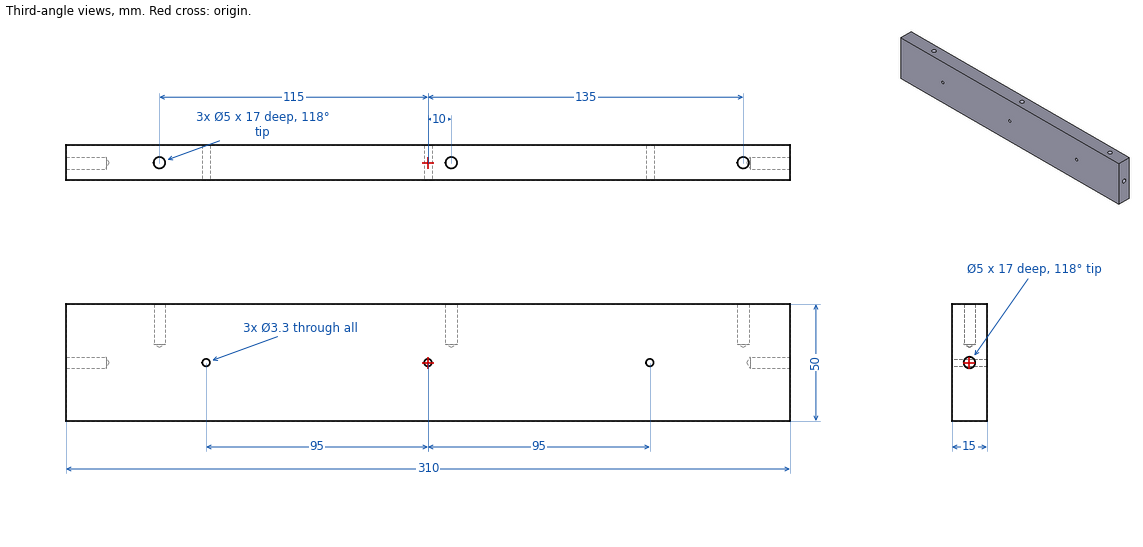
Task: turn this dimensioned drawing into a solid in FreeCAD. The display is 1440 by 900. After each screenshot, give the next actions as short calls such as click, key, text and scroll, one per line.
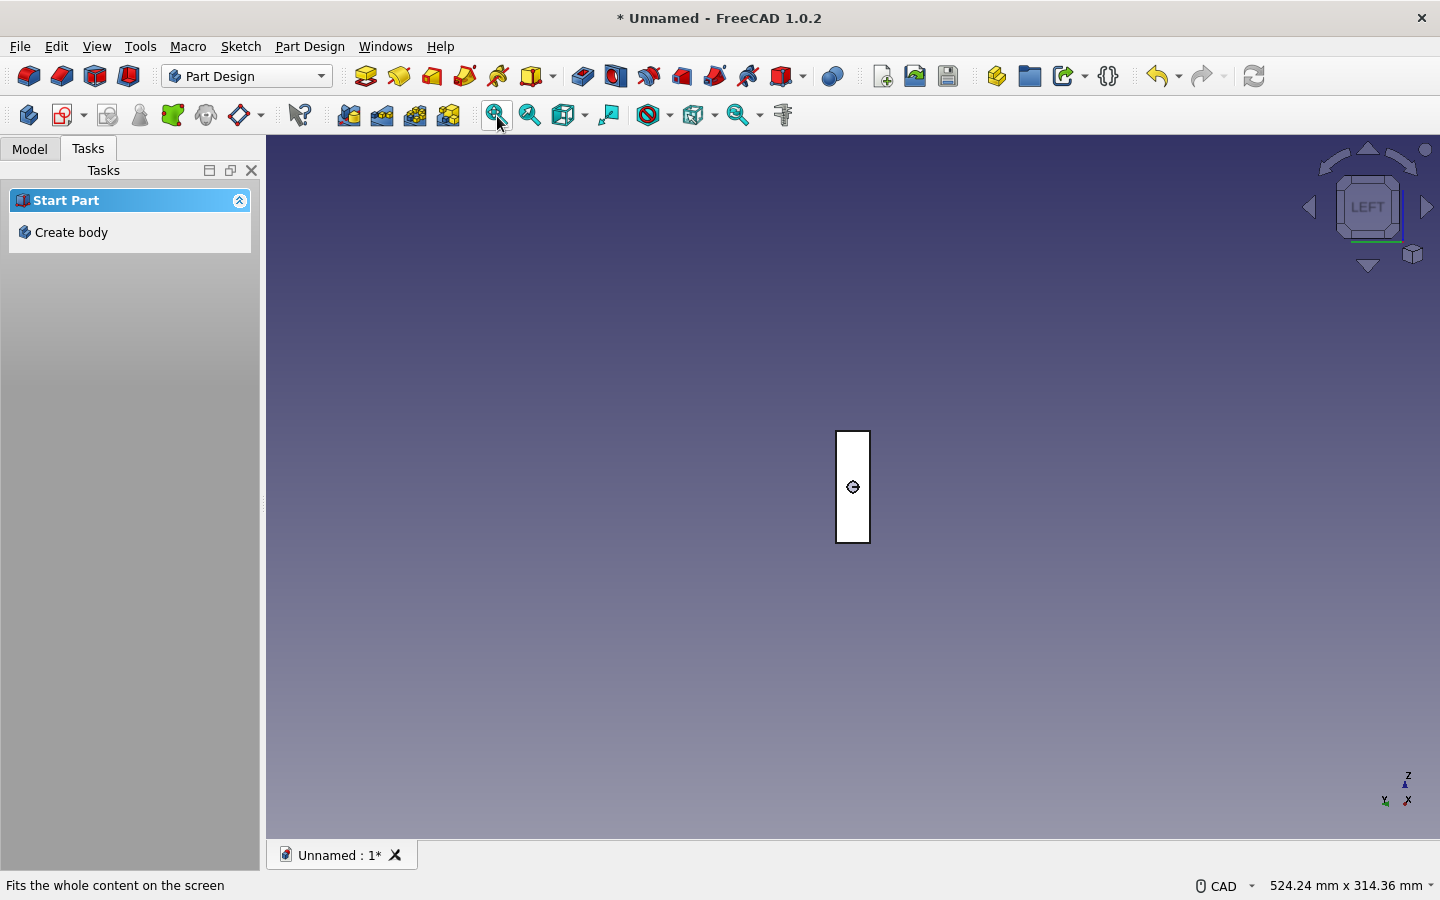
key(4)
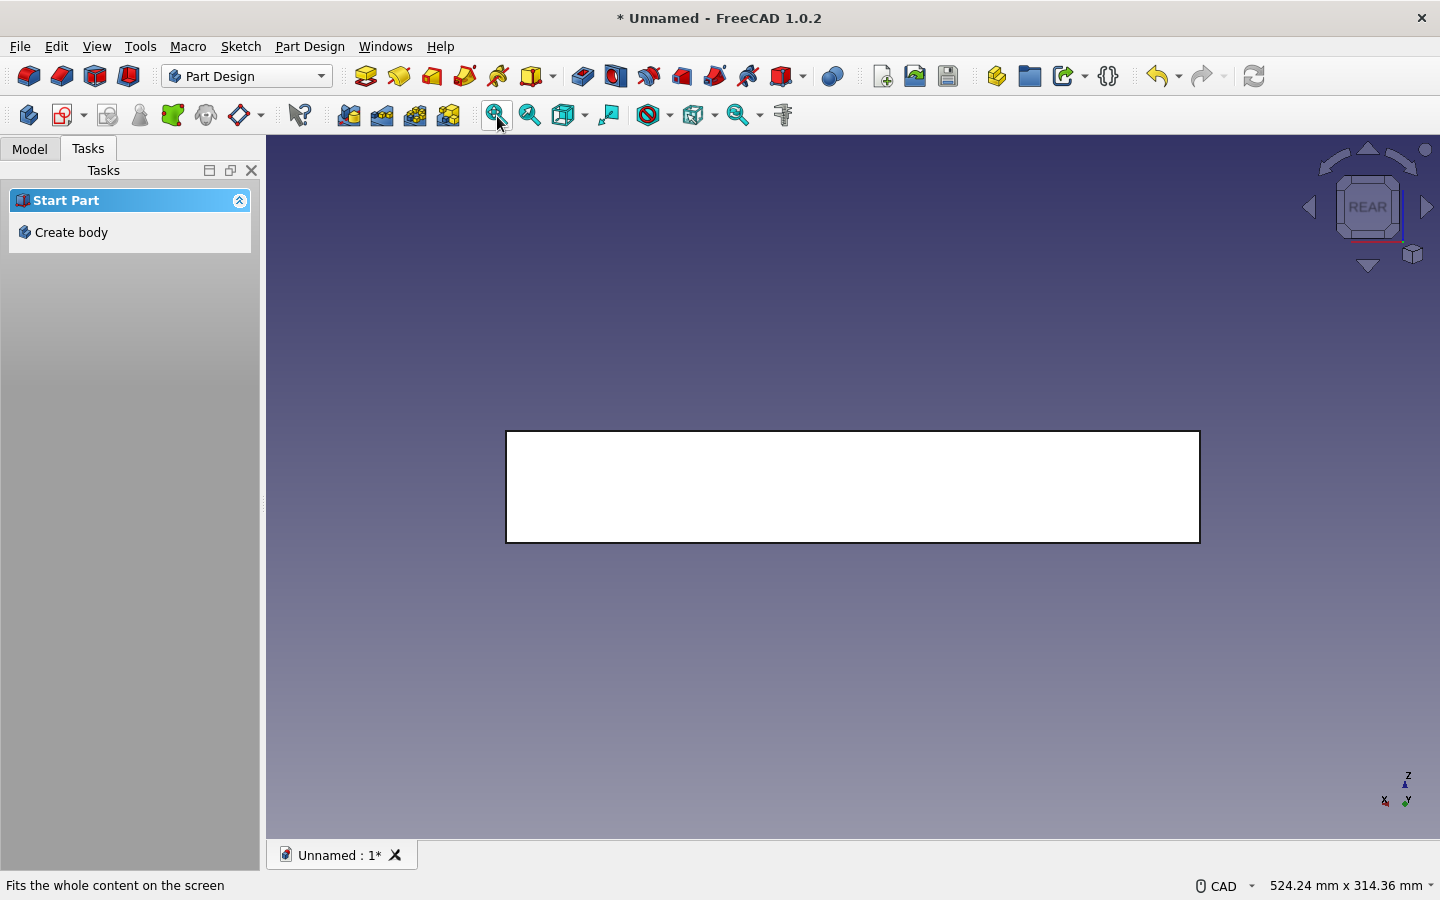
click(655, 486)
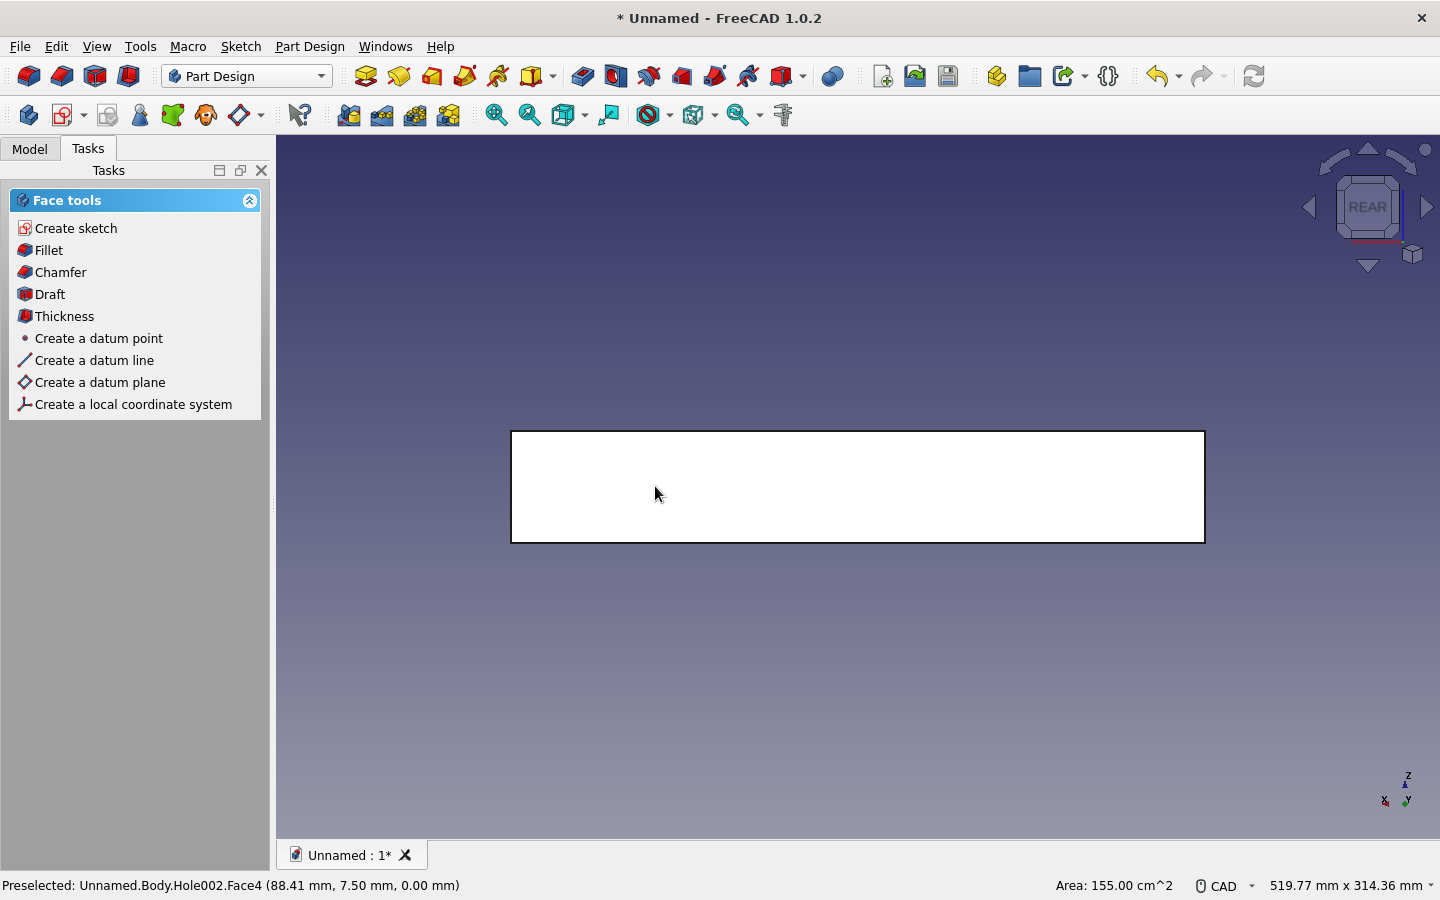
click(62, 116)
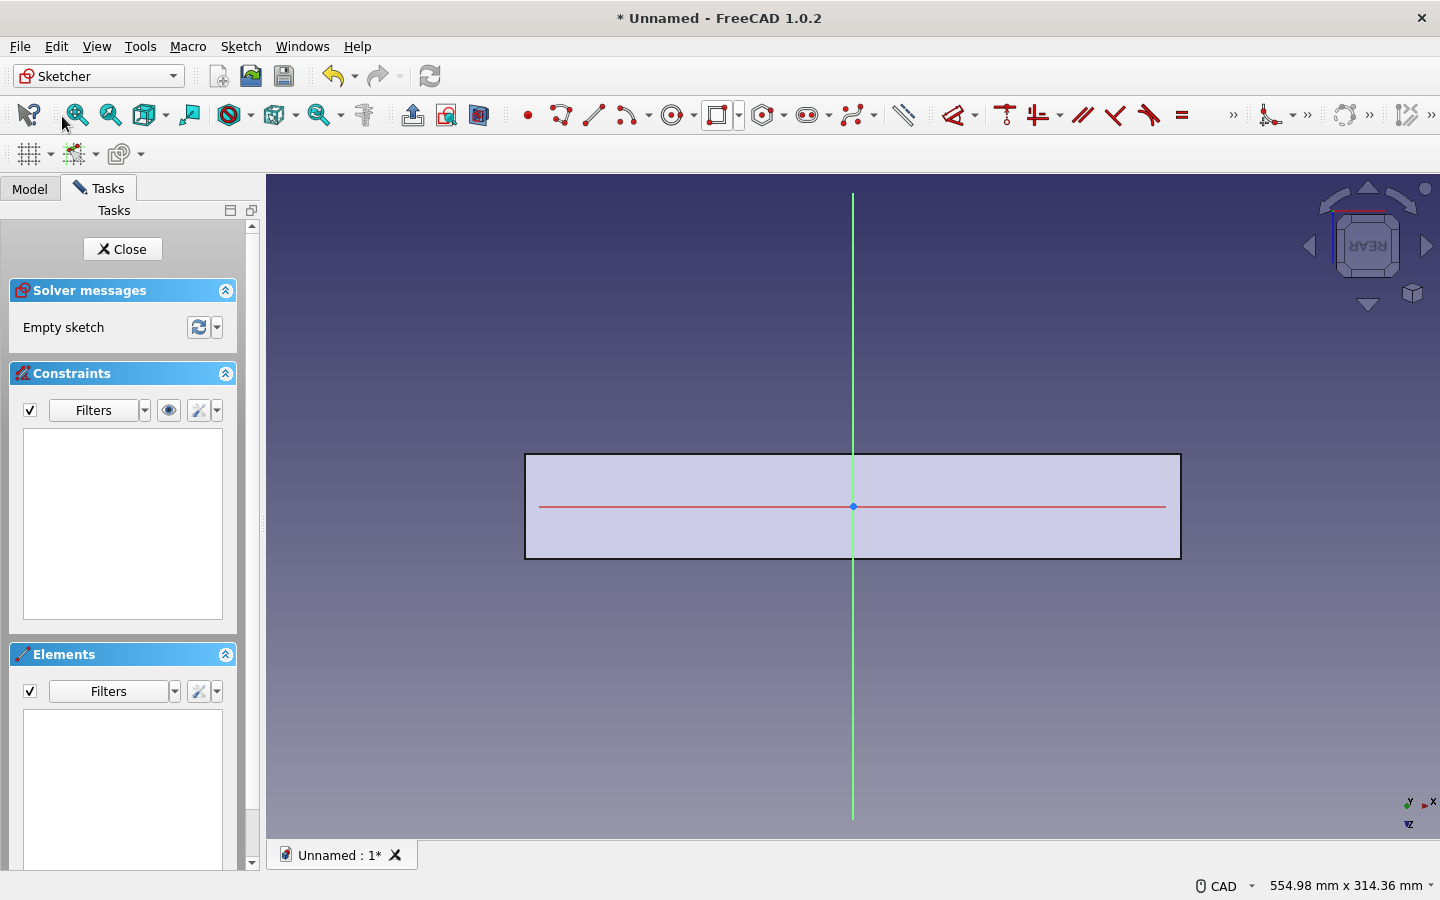
scroll(936, 507, up, 3)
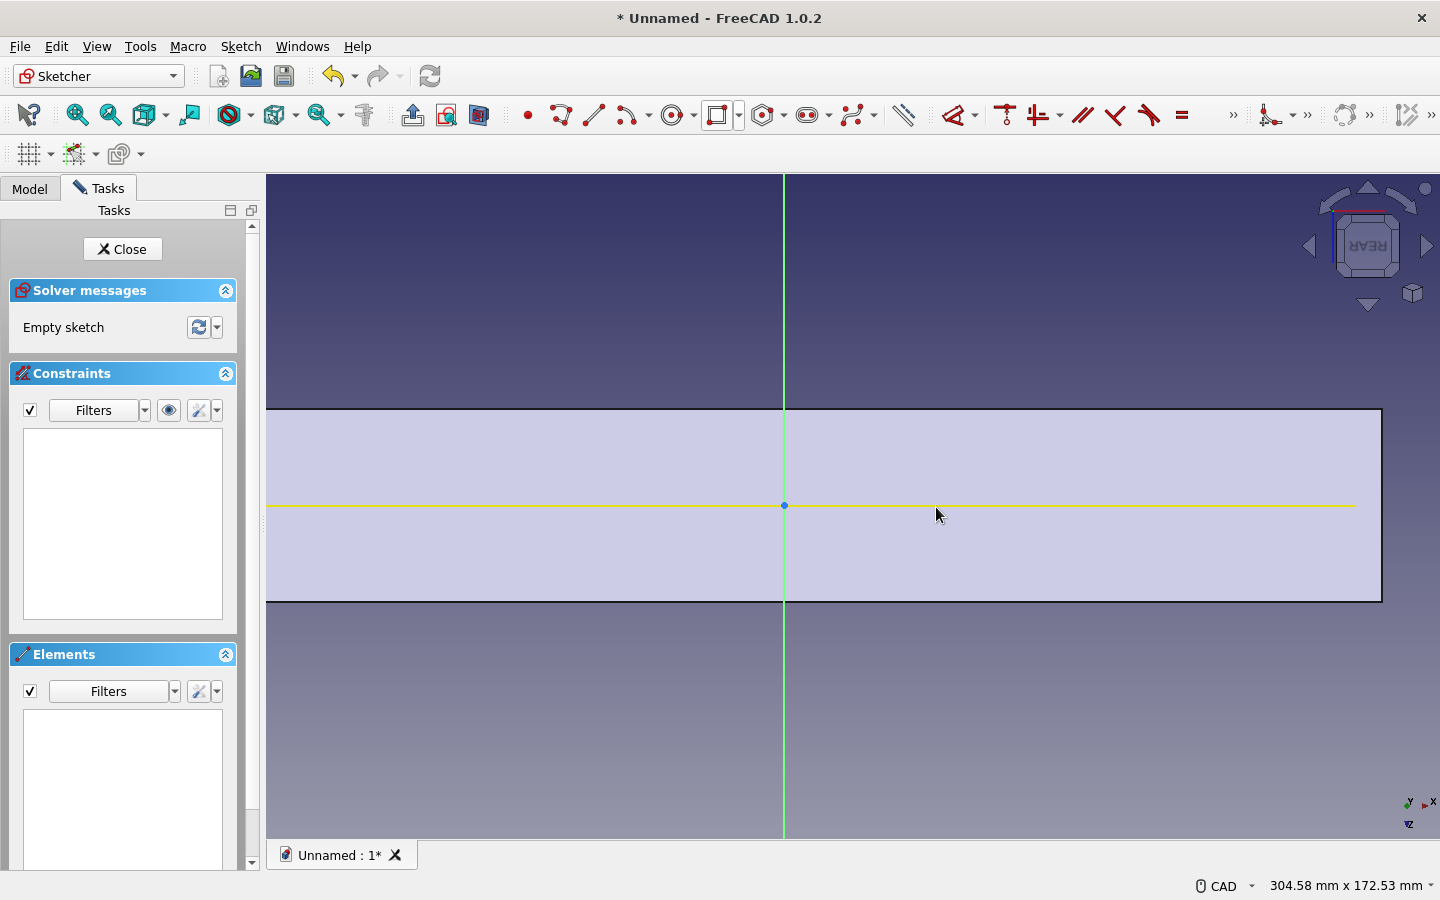
click(672, 116)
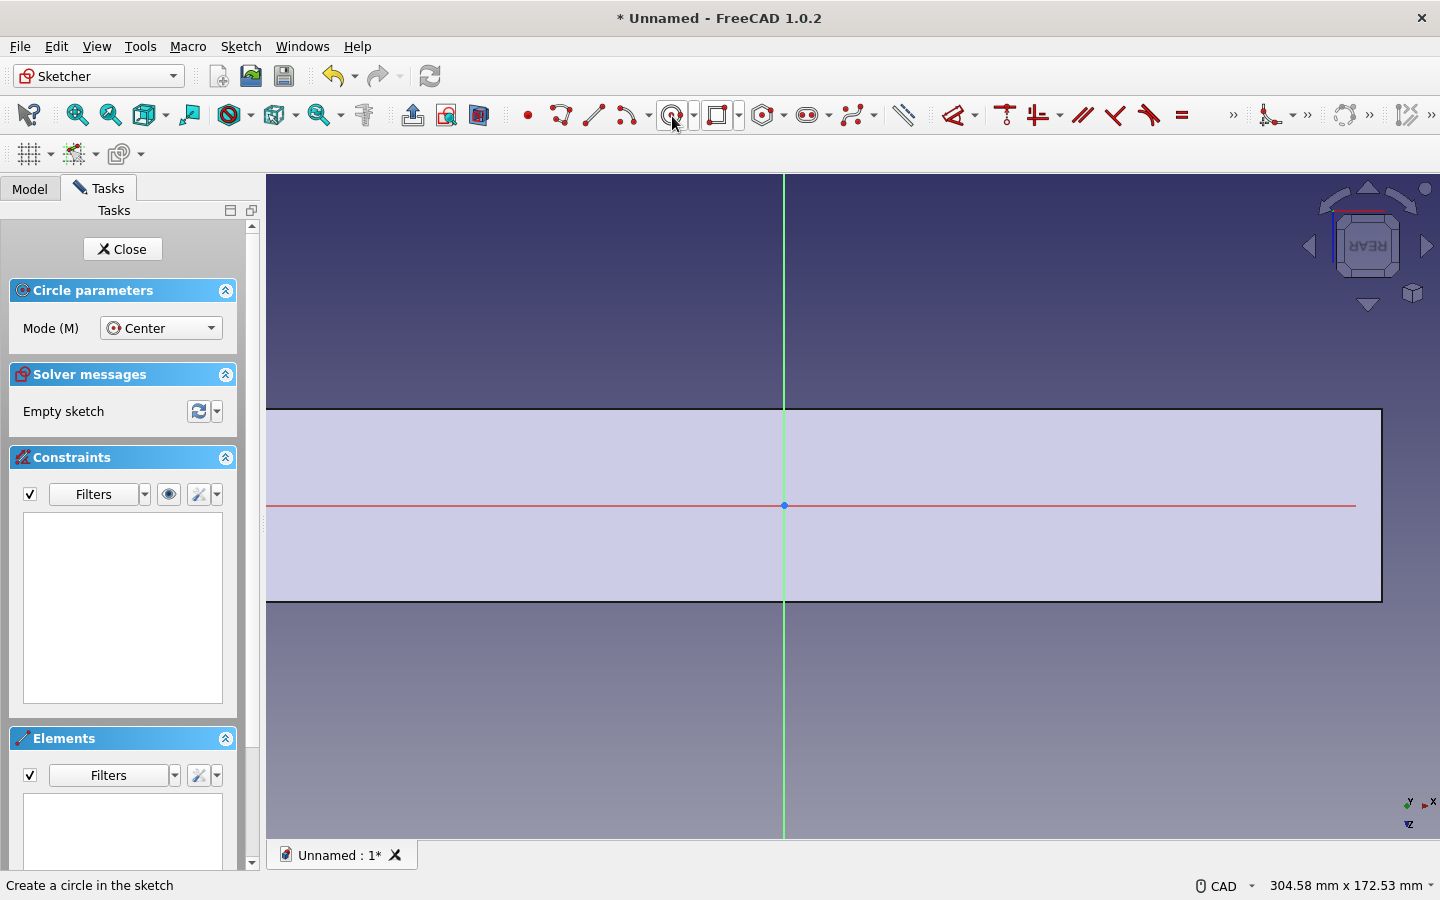
scroll(418, 506, up, 7)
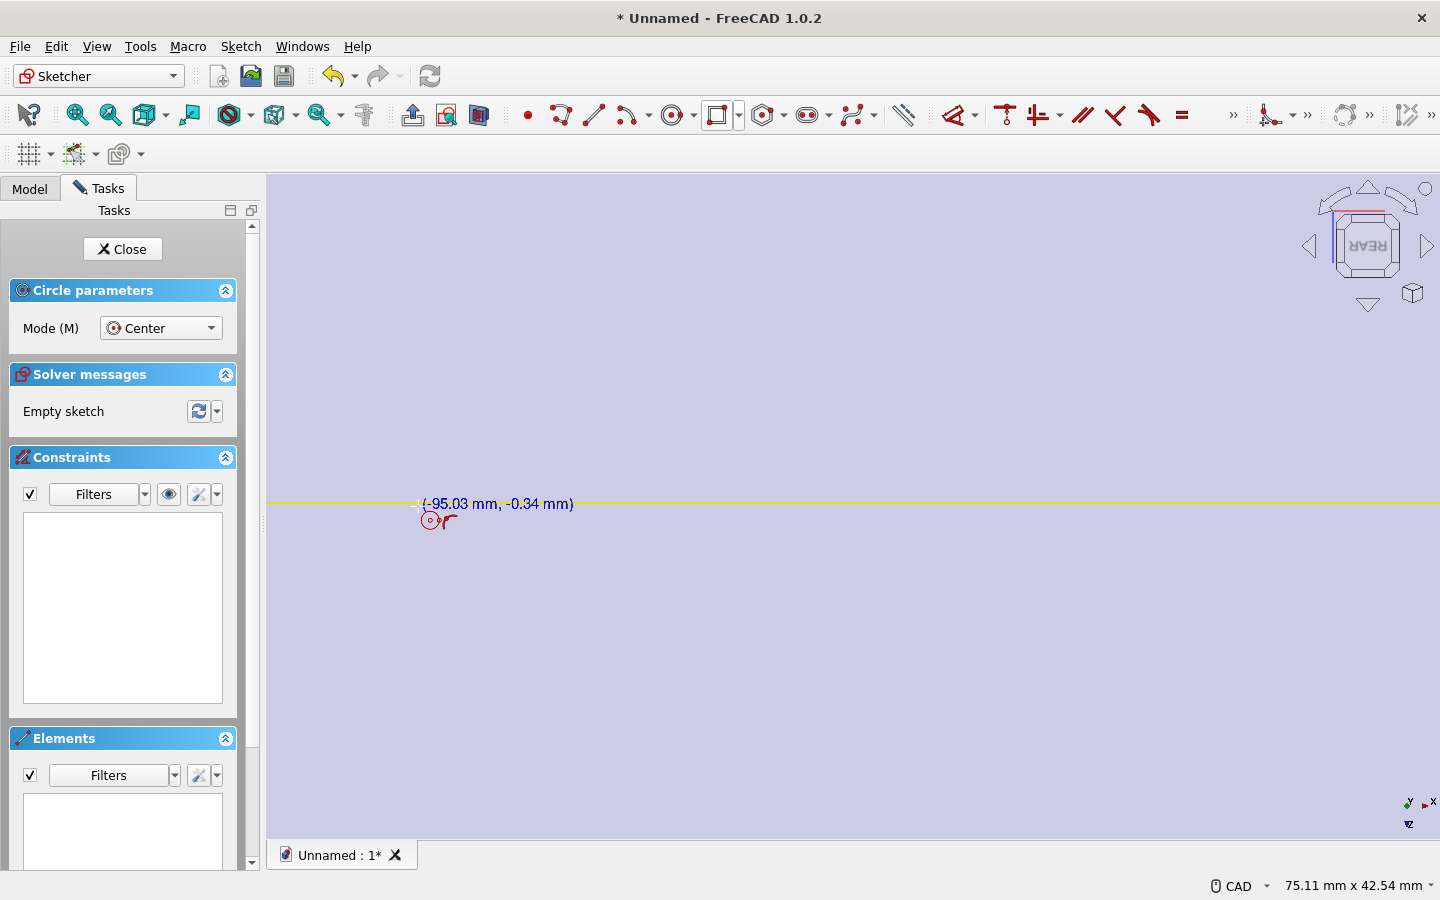
scroll(418, 508, down, 7)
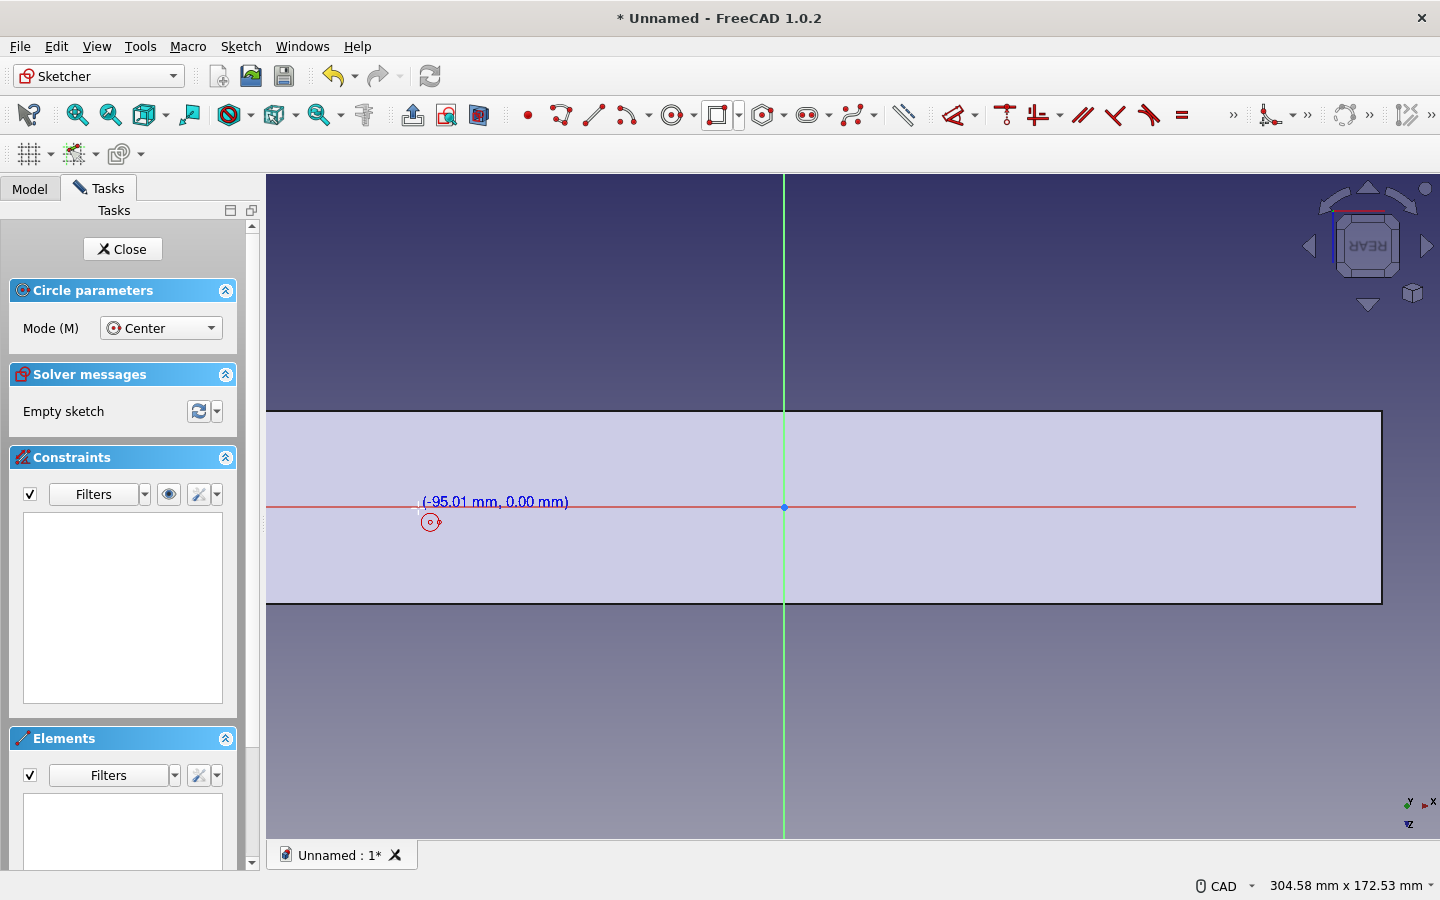
click(418, 507)